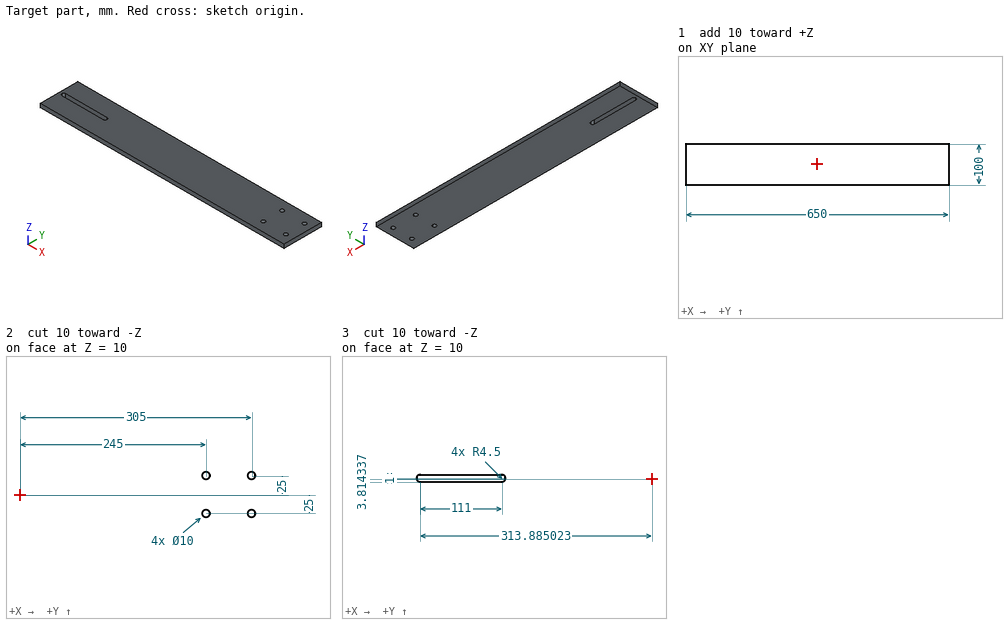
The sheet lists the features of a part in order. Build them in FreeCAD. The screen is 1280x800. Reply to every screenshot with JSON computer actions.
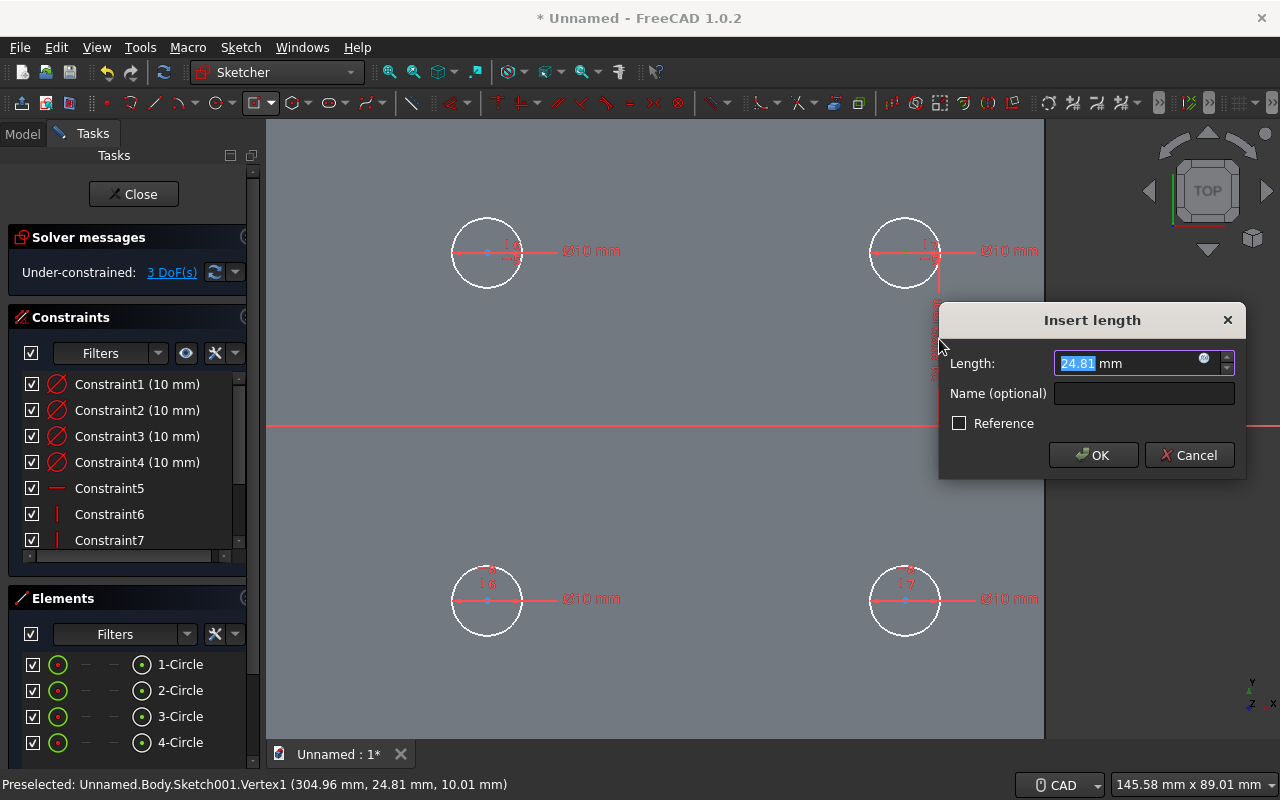
{"action": "type", "text": "25"}
{"action": "key", "text": "Return"}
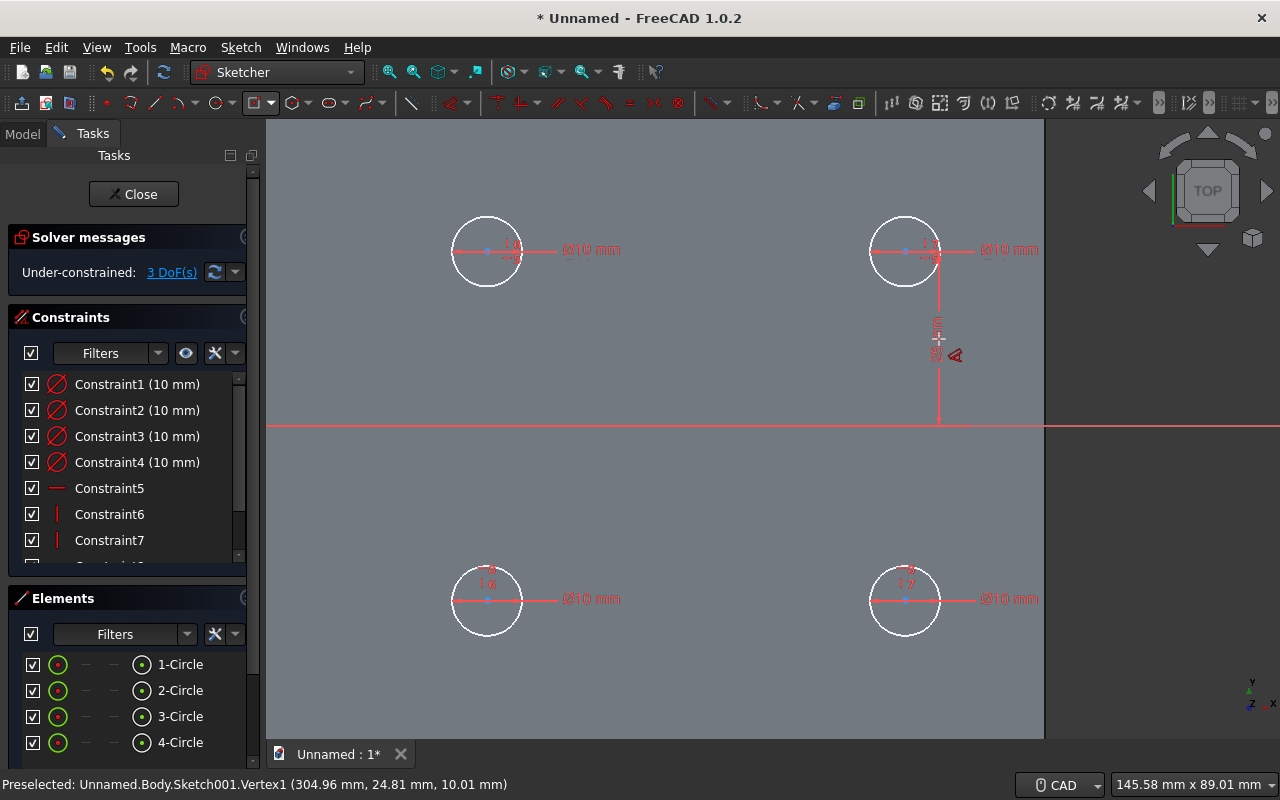
{"action": "left_click", "coordinate": [487, 601]}
{"action": "left_click", "coordinate": [521, 513]}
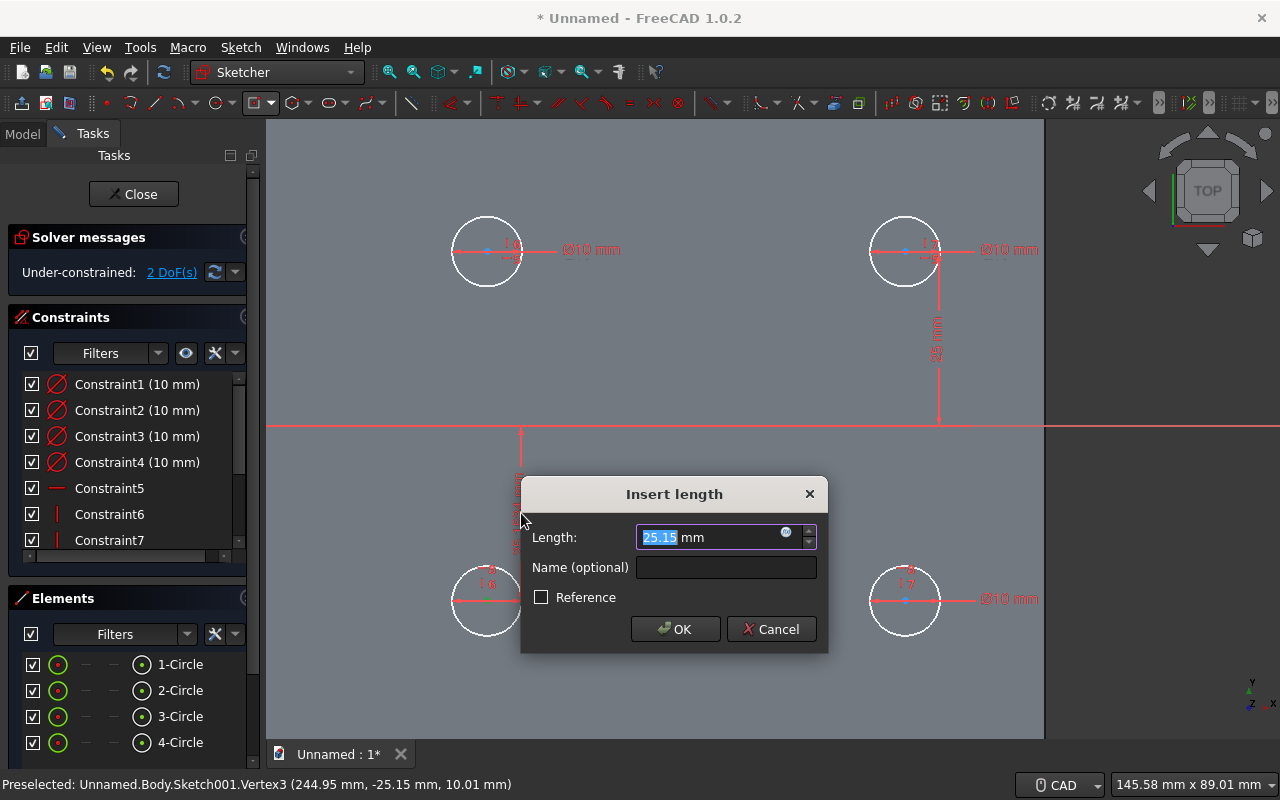
{"action": "type", "text": "25"}
{"action": "key", "text": "Return"}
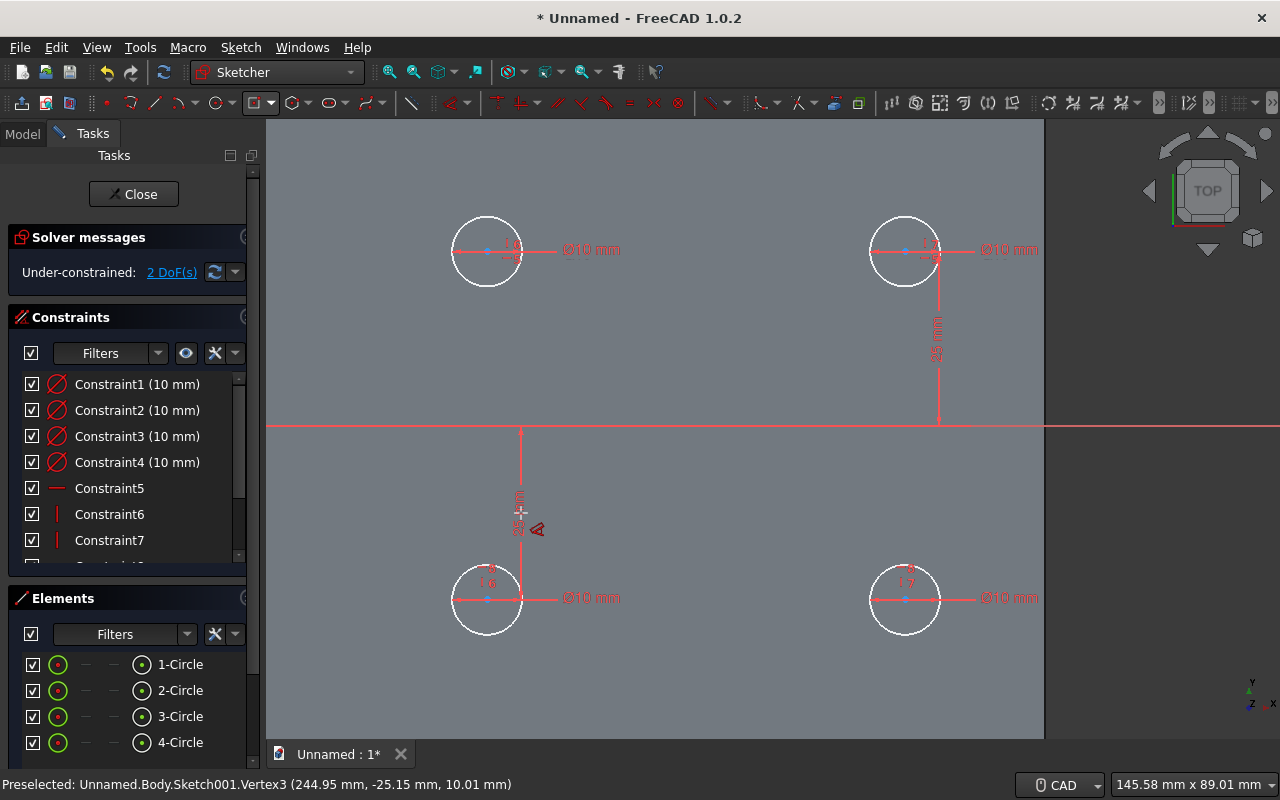
{"action": "left_click", "coordinate": [905, 252]}
{"action": "left_click", "coordinate": [600, 218]}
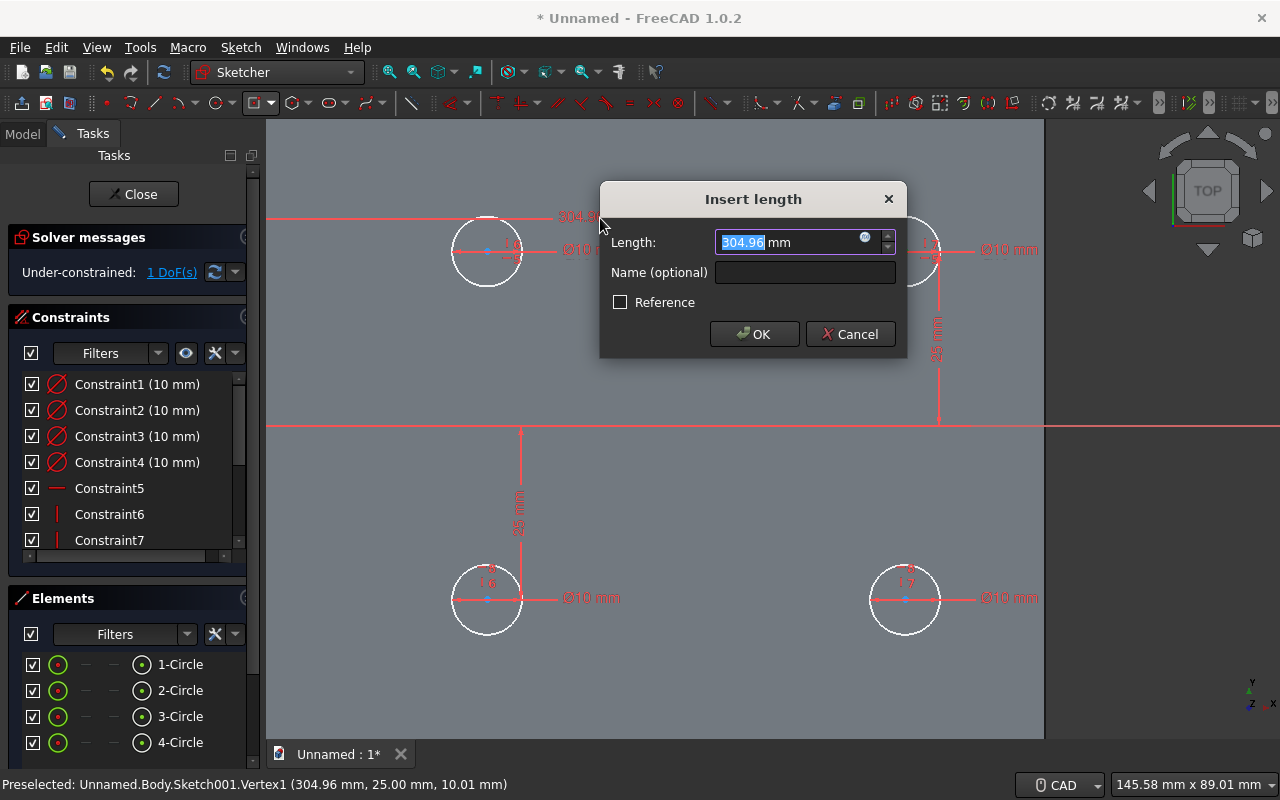
{"action": "type", "text": "305"}
{"action": "key", "text": "Return"}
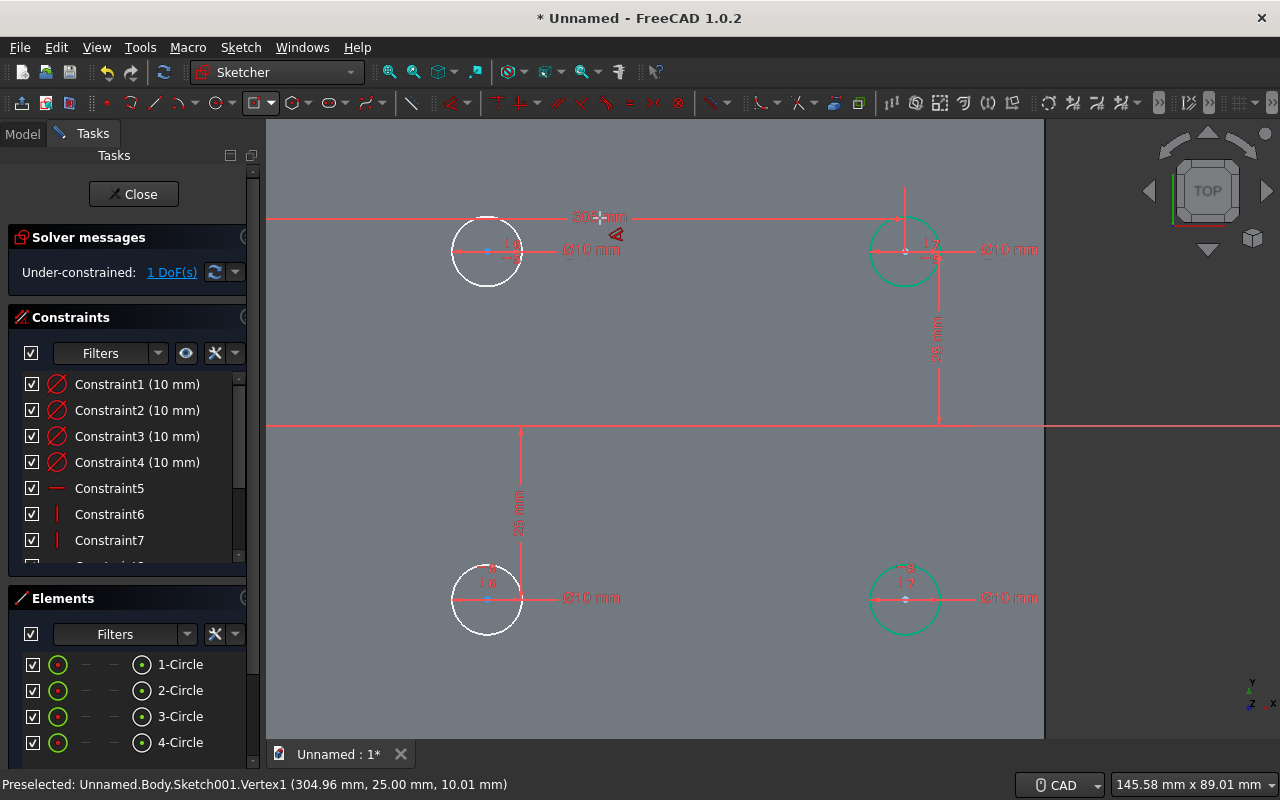
{"action": "left_click", "coordinate": [487, 252]}
{"action": "left_click", "coordinate": [390, 218]}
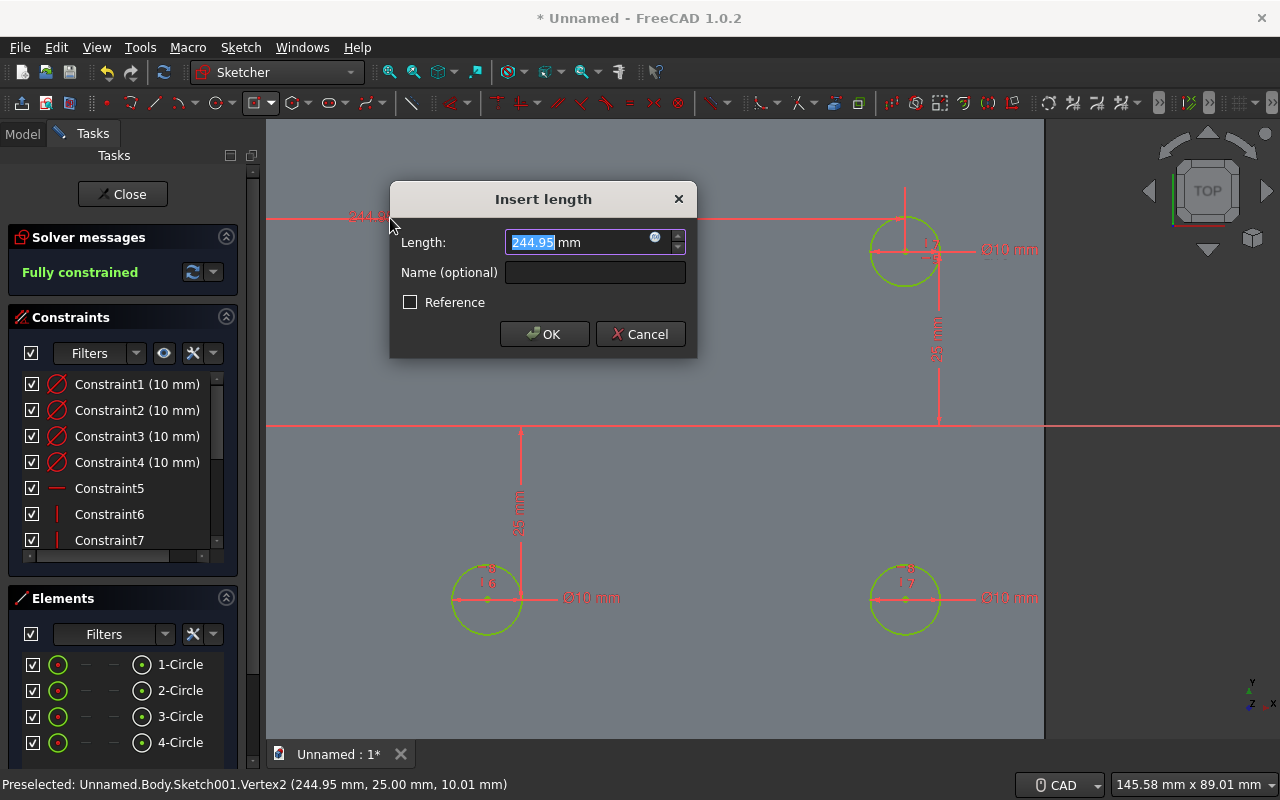
{"action": "type", "text": "245"}
{"action": "key", "text": "Return"}
{"action": "key", "text": "Escape"}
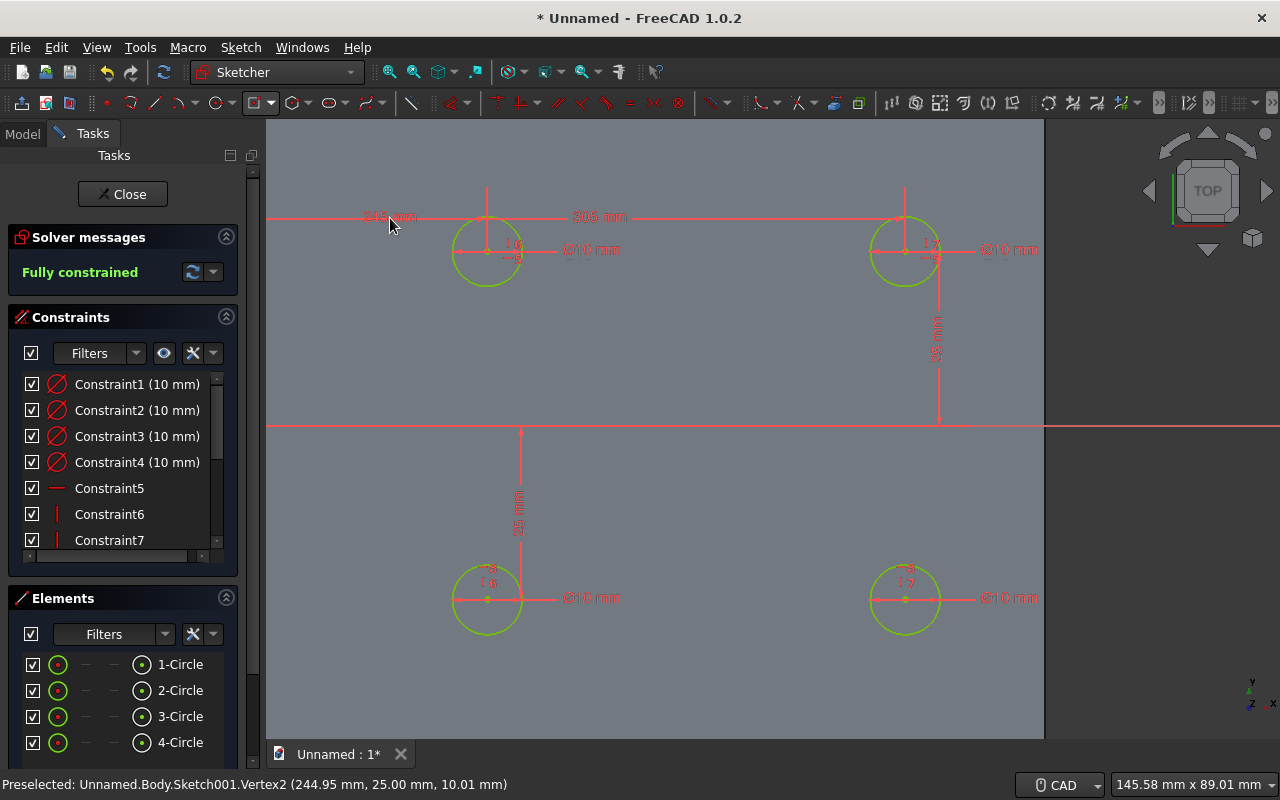
{"action": "left_click", "coordinate": [123, 194]}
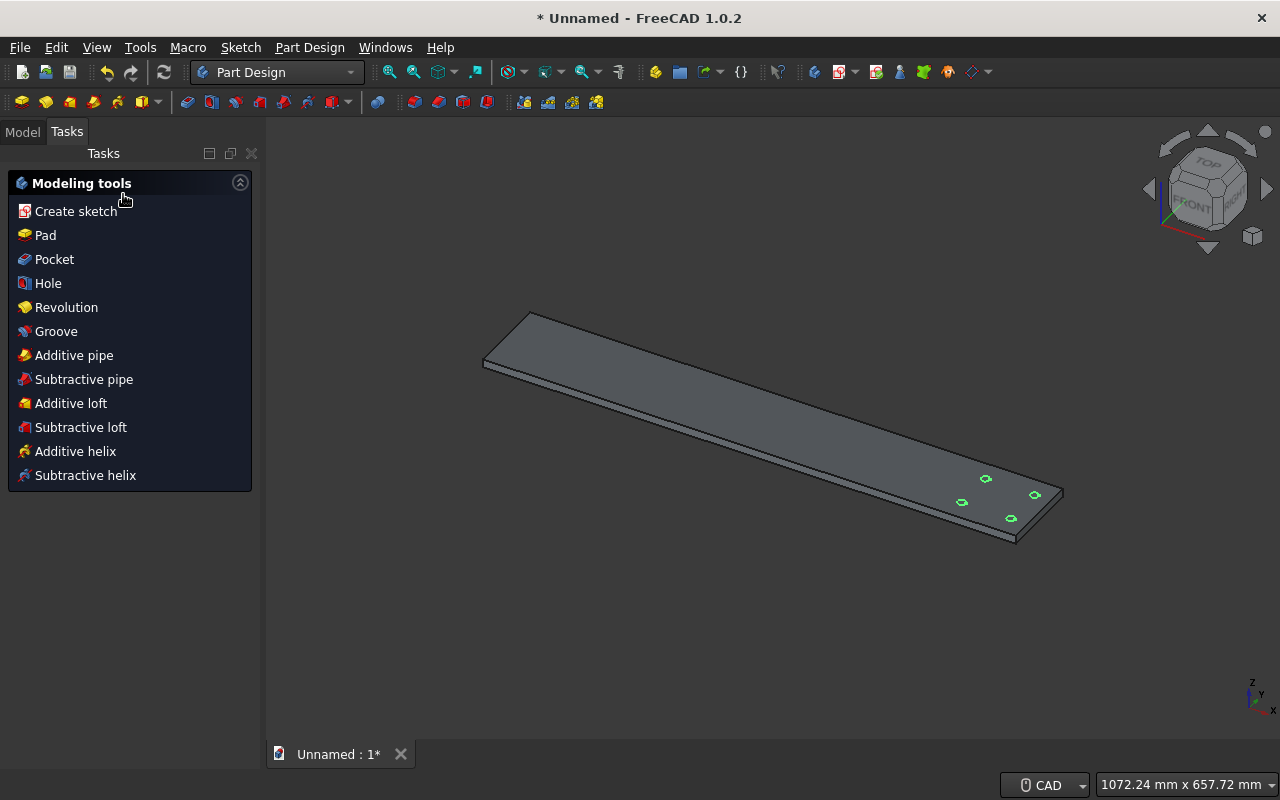
{"action": "left_click", "coordinate": [188, 102]}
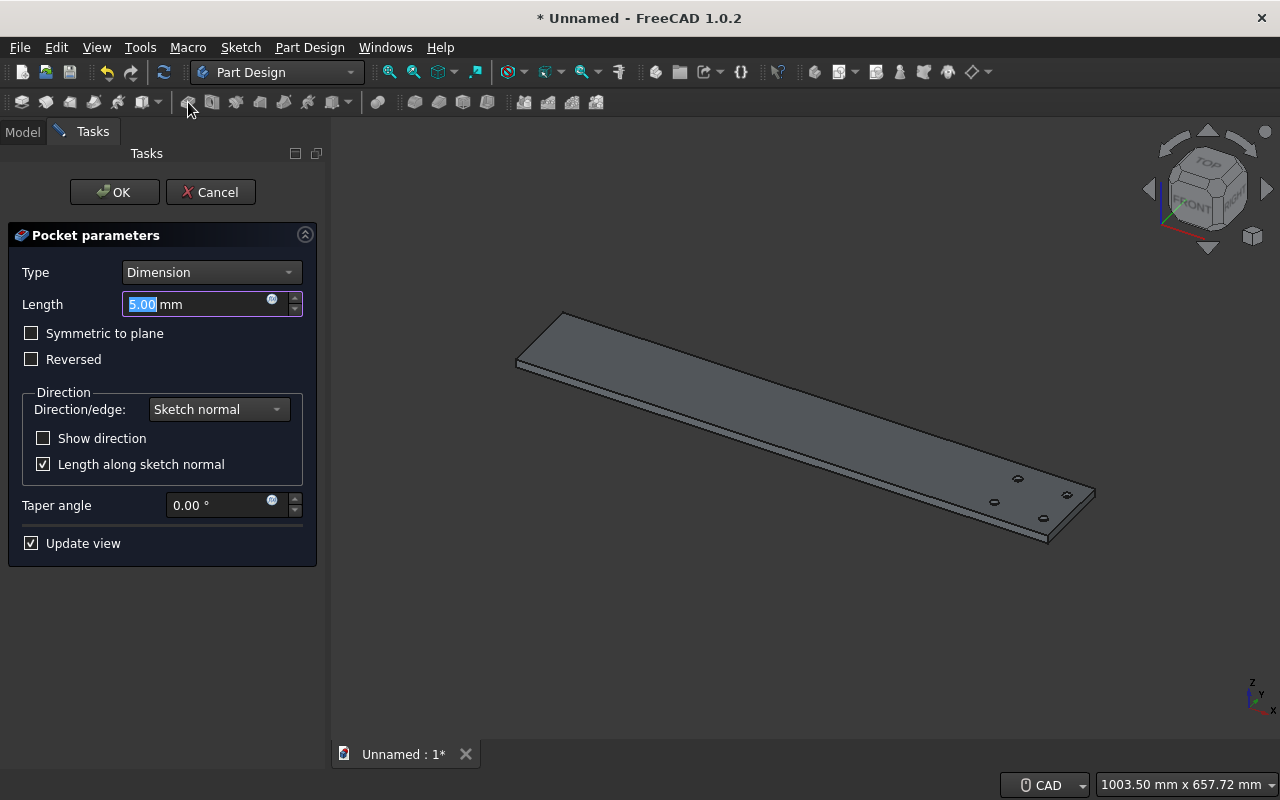
{"action": "type", "text": "10"}
{"action": "key", "text": "Tab"}